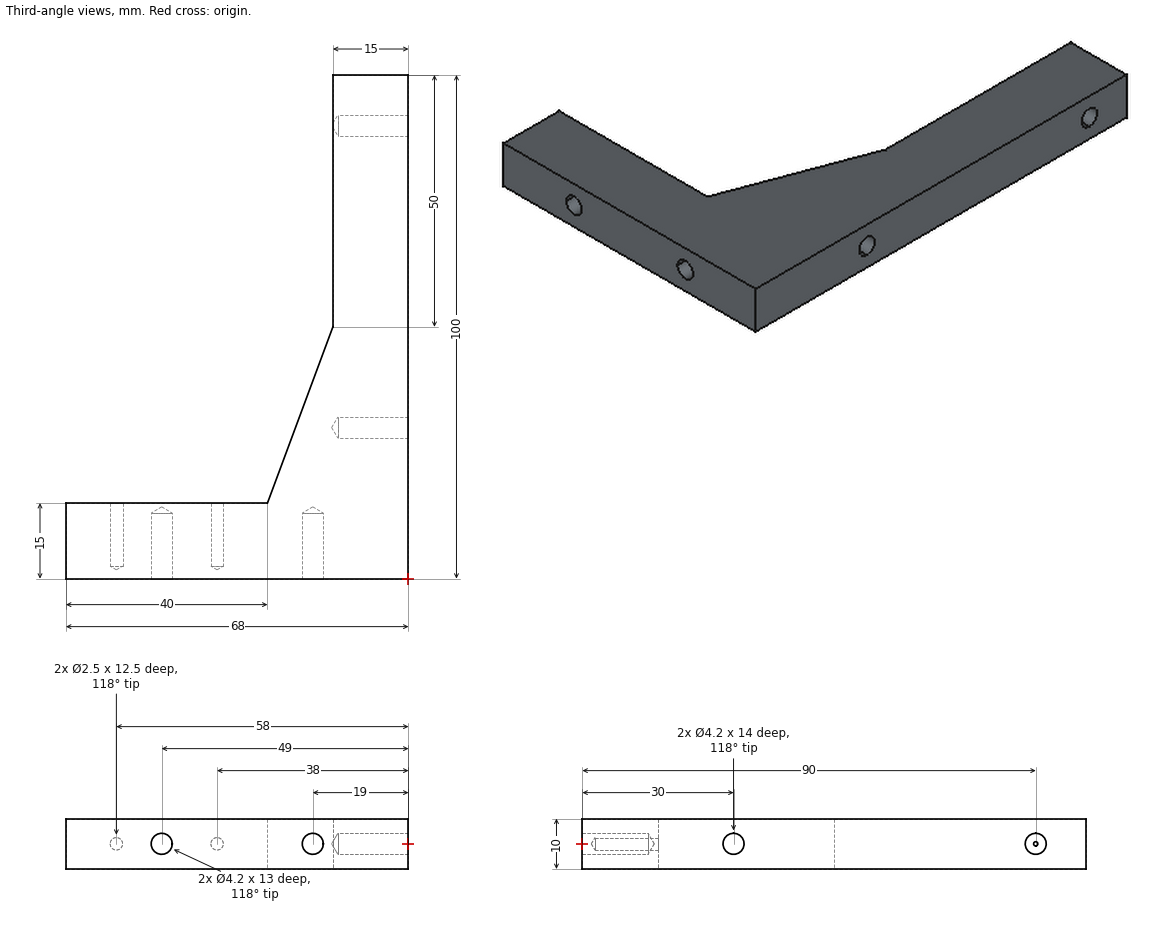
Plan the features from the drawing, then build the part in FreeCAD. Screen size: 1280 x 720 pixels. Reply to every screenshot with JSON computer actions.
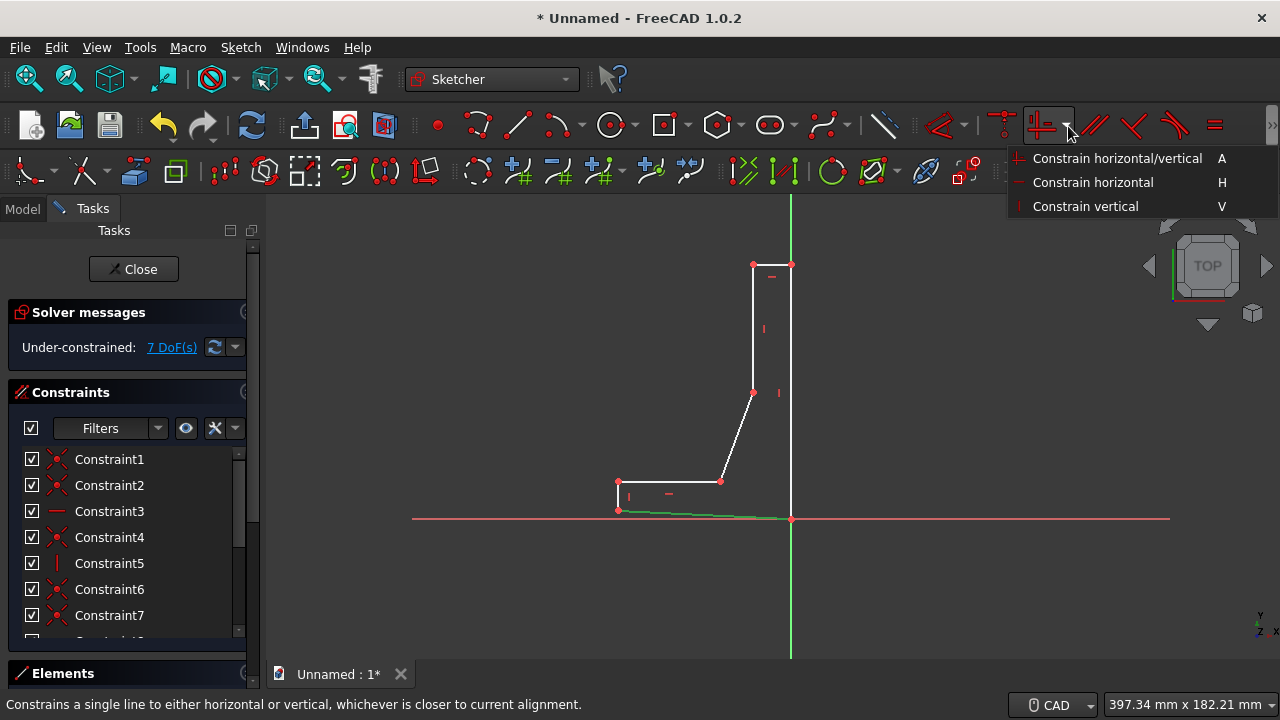
{"action": "left_click", "coordinate": [1143, 182]}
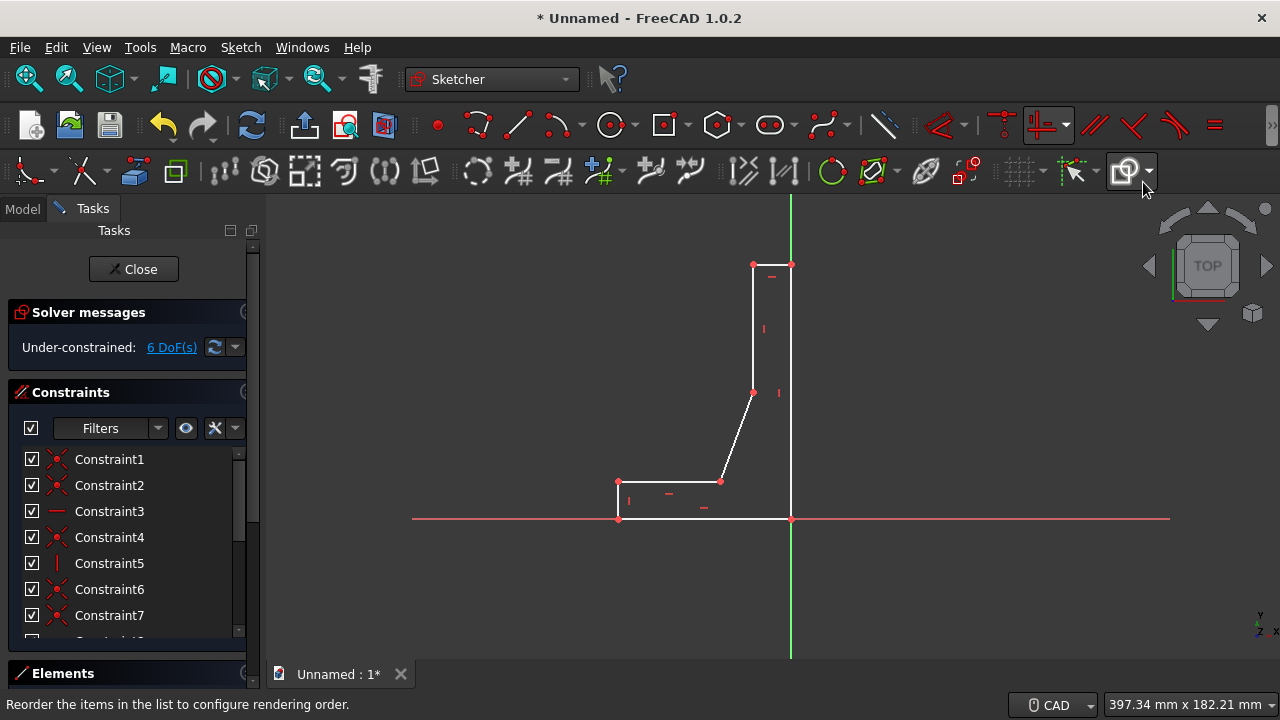
{"action": "key", "text": "d"}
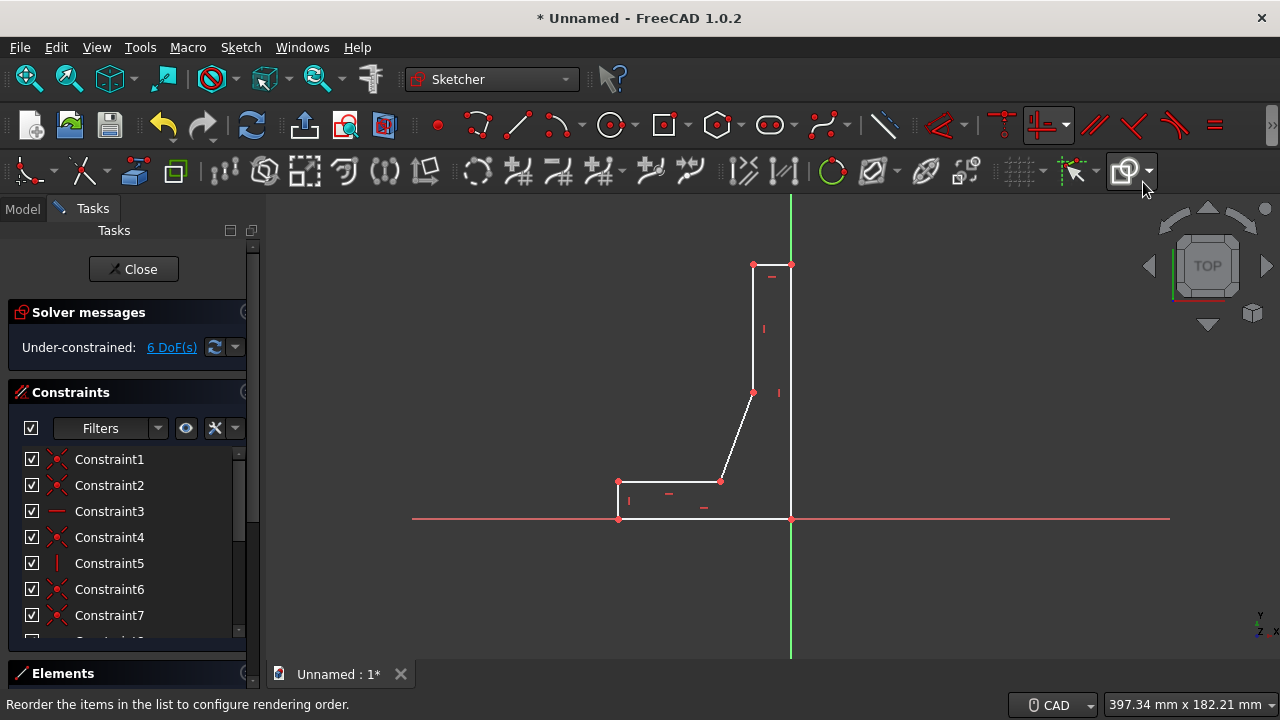
{"action": "left_click", "coordinate": [780, 265]}
{"action": "left_click", "coordinate": [772, 231]}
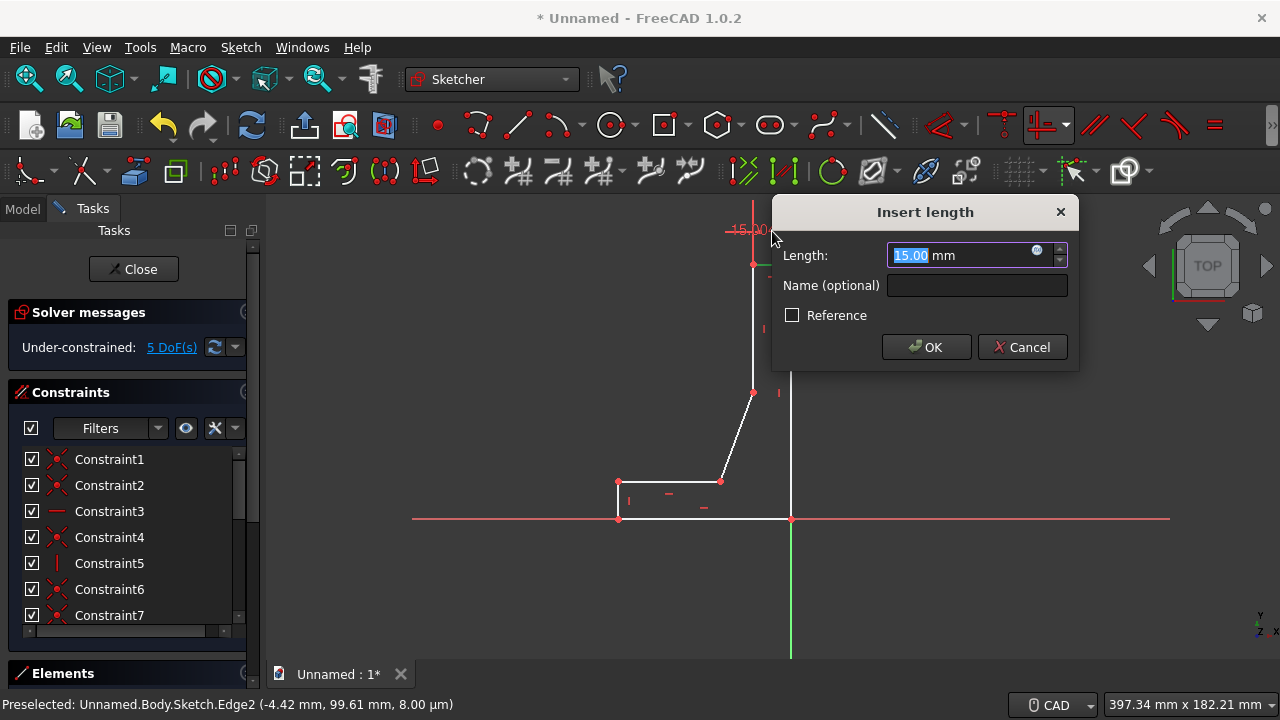
{"action": "type", "text": "15"}
{"action": "key", "text": "Return"}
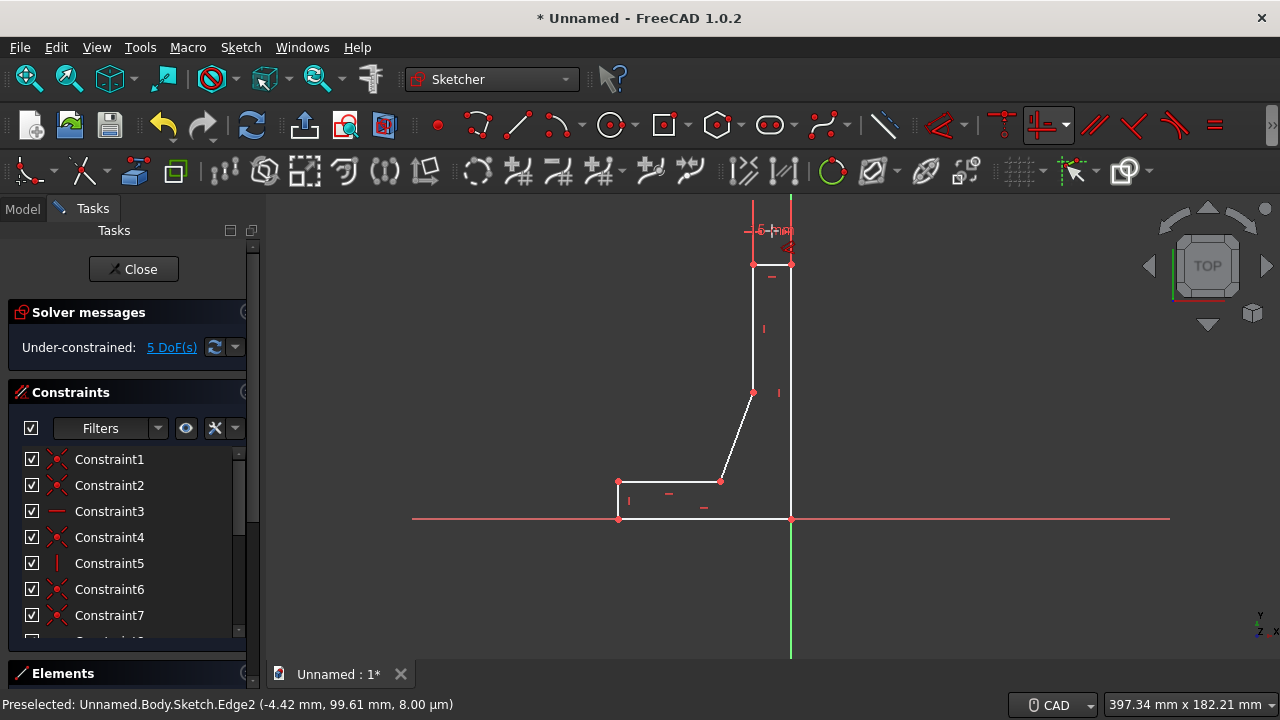
{"action": "left_click", "coordinate": [753, 303]}
{"action": "left_click", "coordinate": [719, 329]}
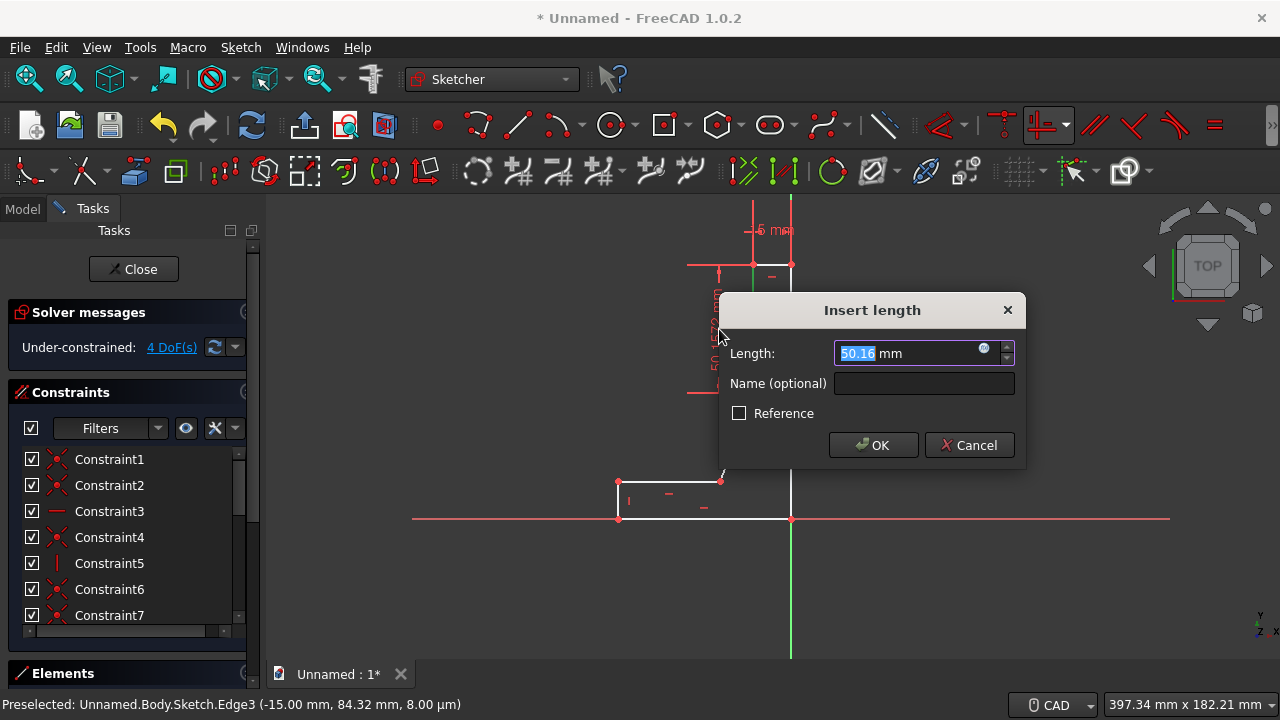
{"action": "type", "text": "50"}
{"action": "key", "text": "Return"}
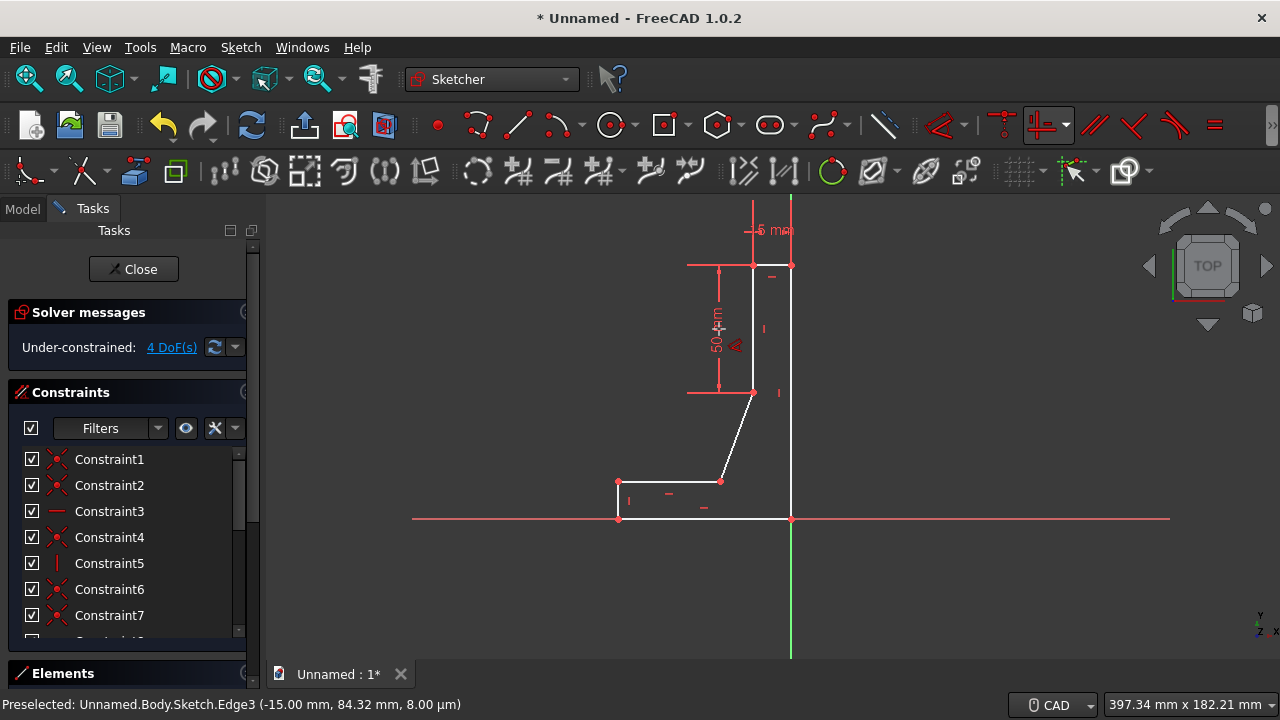
{"action": "left_click", "coordinate": [689, 482]}
{"action": "left_click", "coordinate": [669, 448]}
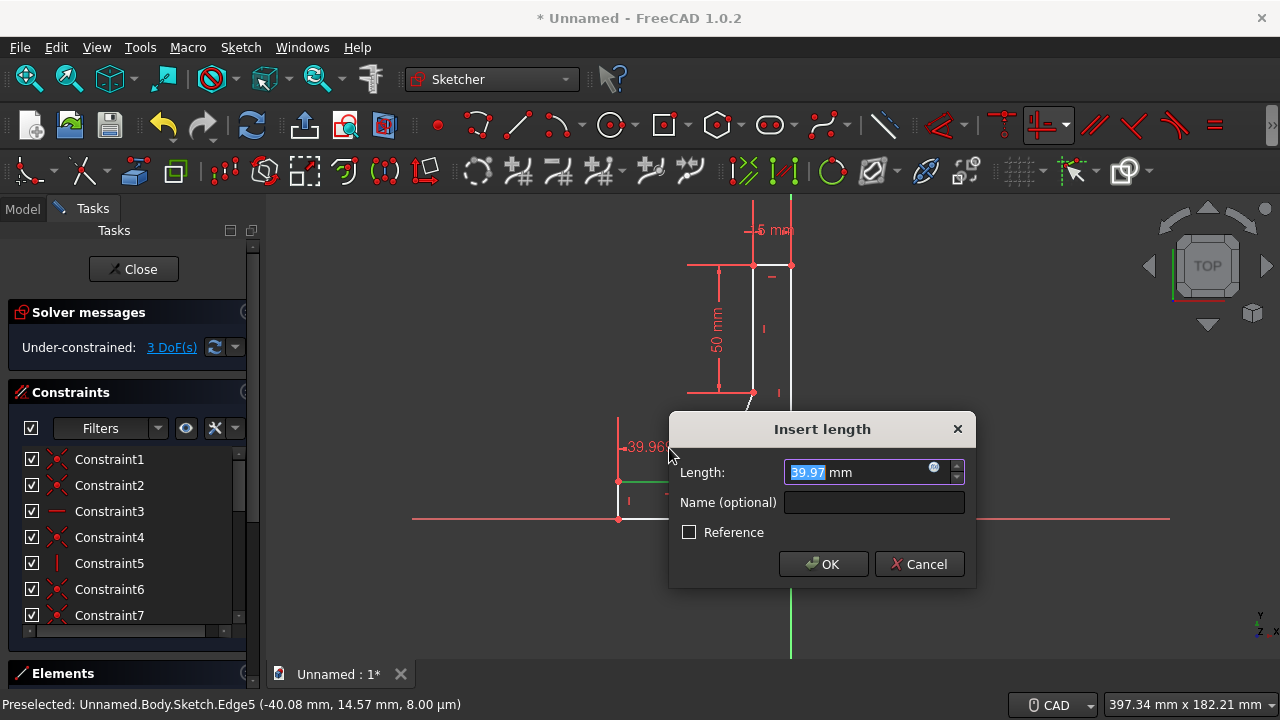
{"action": "type", "text": "40"}
{"action": "key", "text": "Return"}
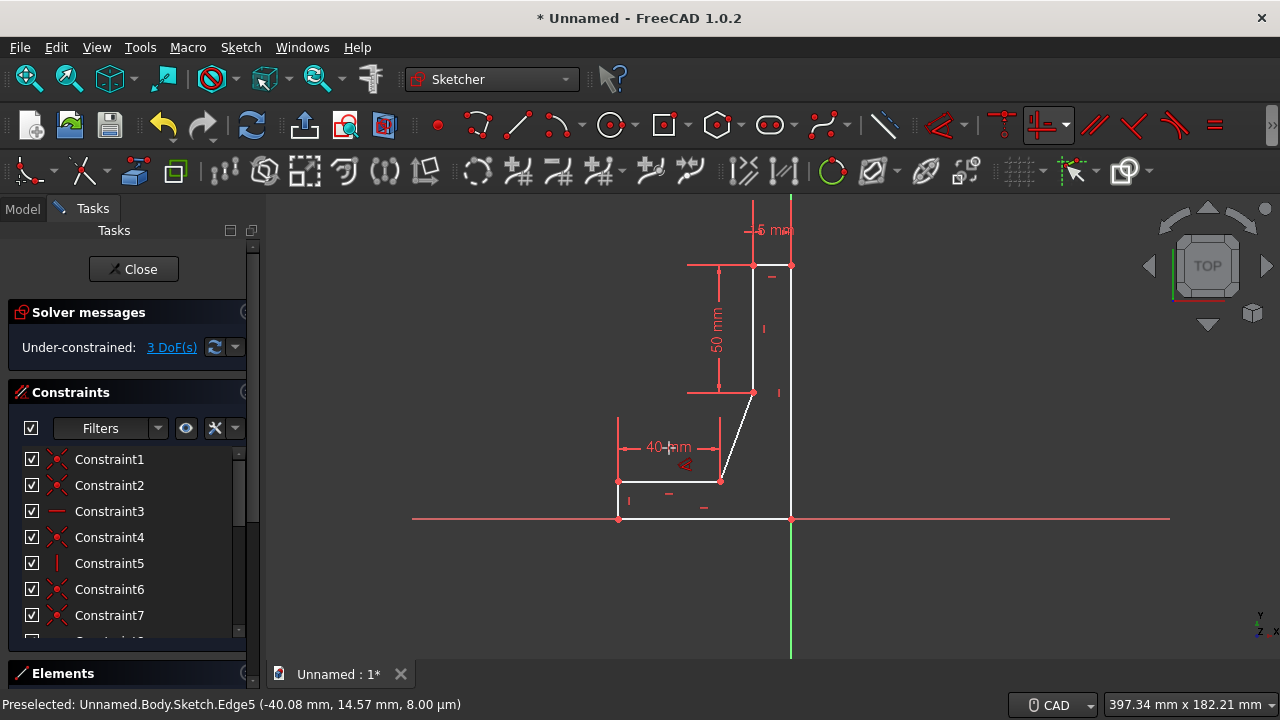
{"action": "scroll", "coordinate": [618, 493], "scroll_direction": "up", "scroll_amount": 2}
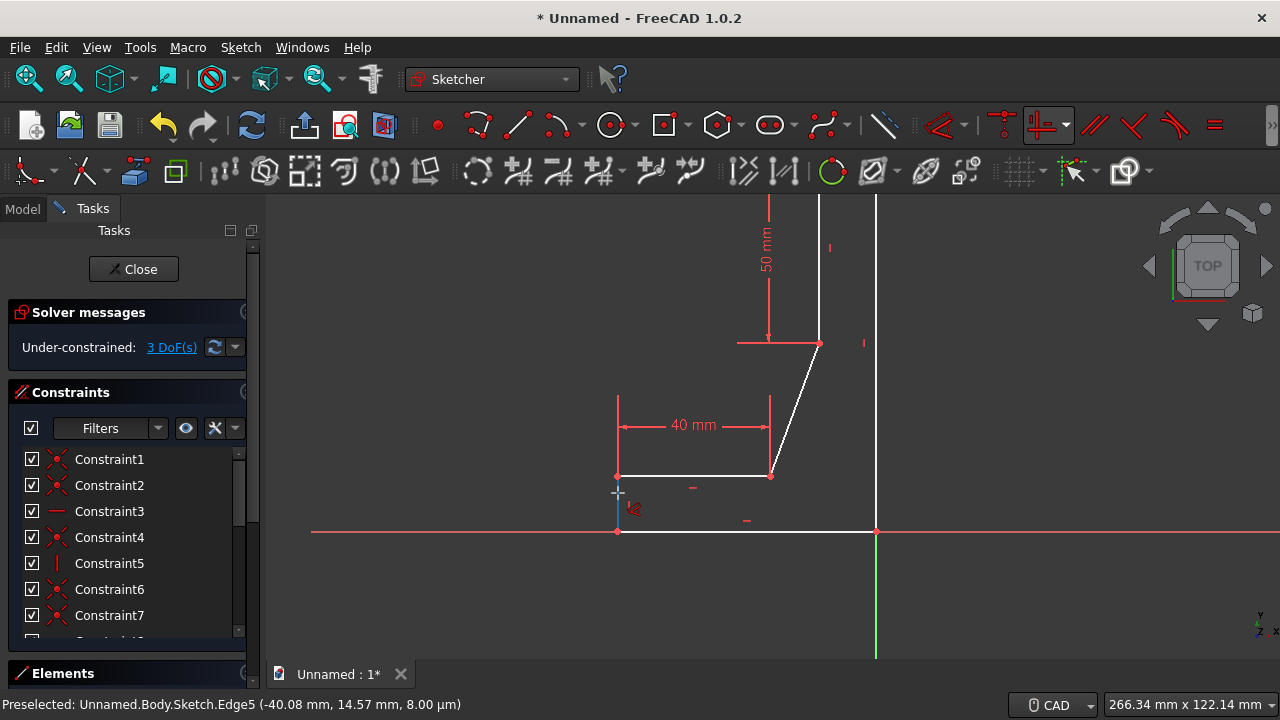
{"action": "left_click", "coordinate": [618, 493]}
{"action": "left_click", "coordinate": [584, 504]}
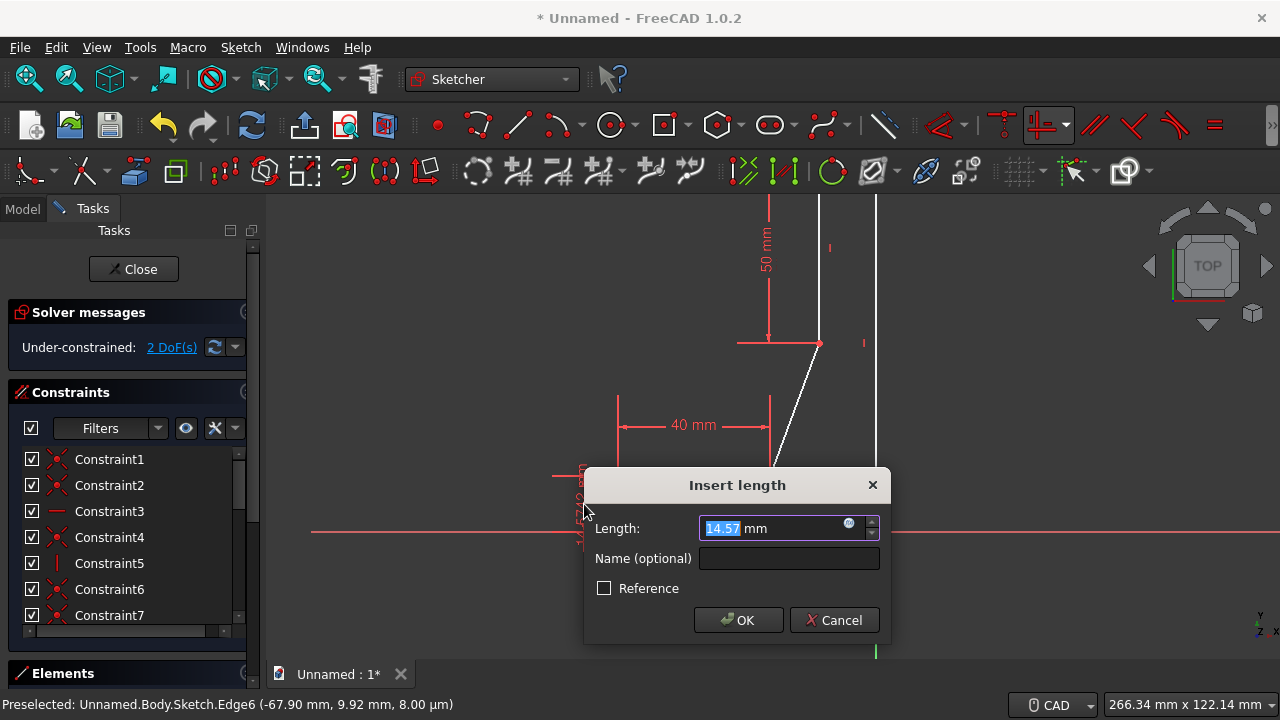
{"action": "type", "text": "15"}
{"action": "key", "text": "Return"}